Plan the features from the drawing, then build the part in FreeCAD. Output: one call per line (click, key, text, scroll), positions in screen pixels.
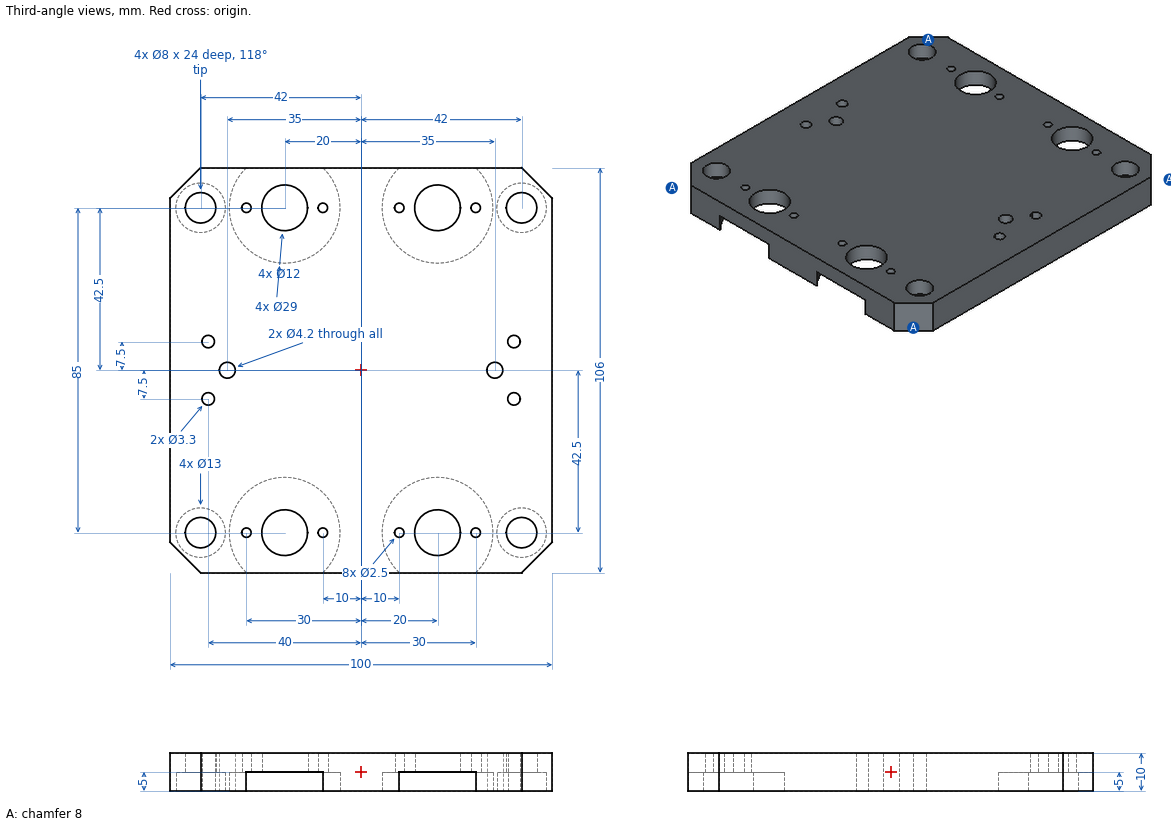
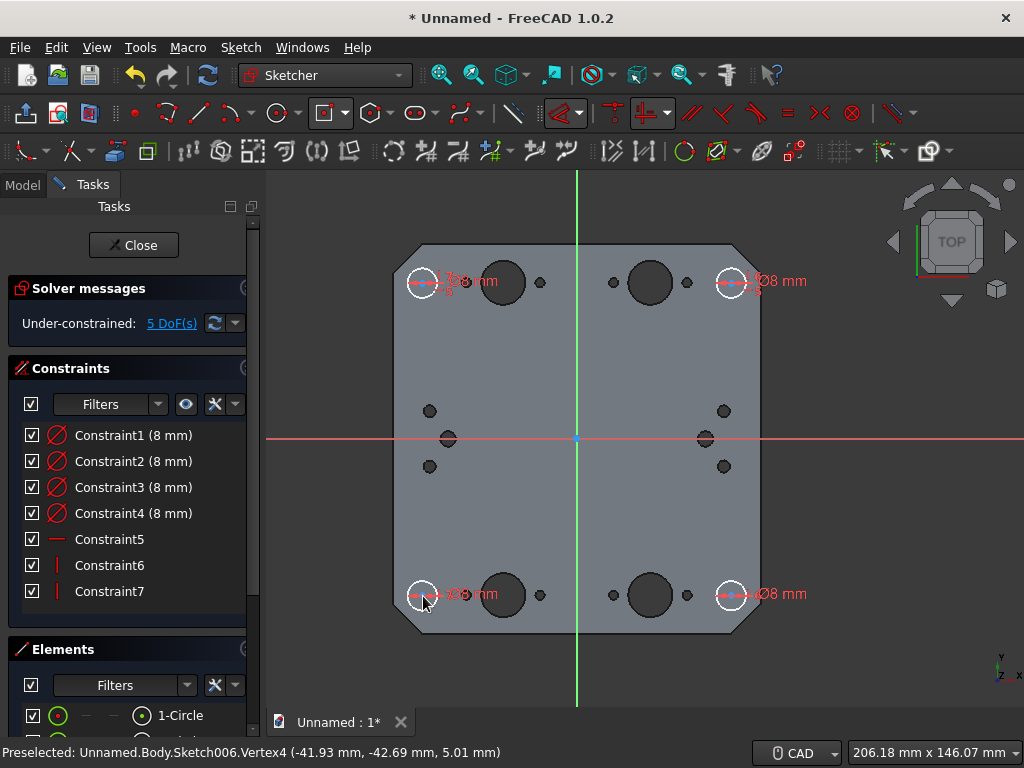
click(731, 596)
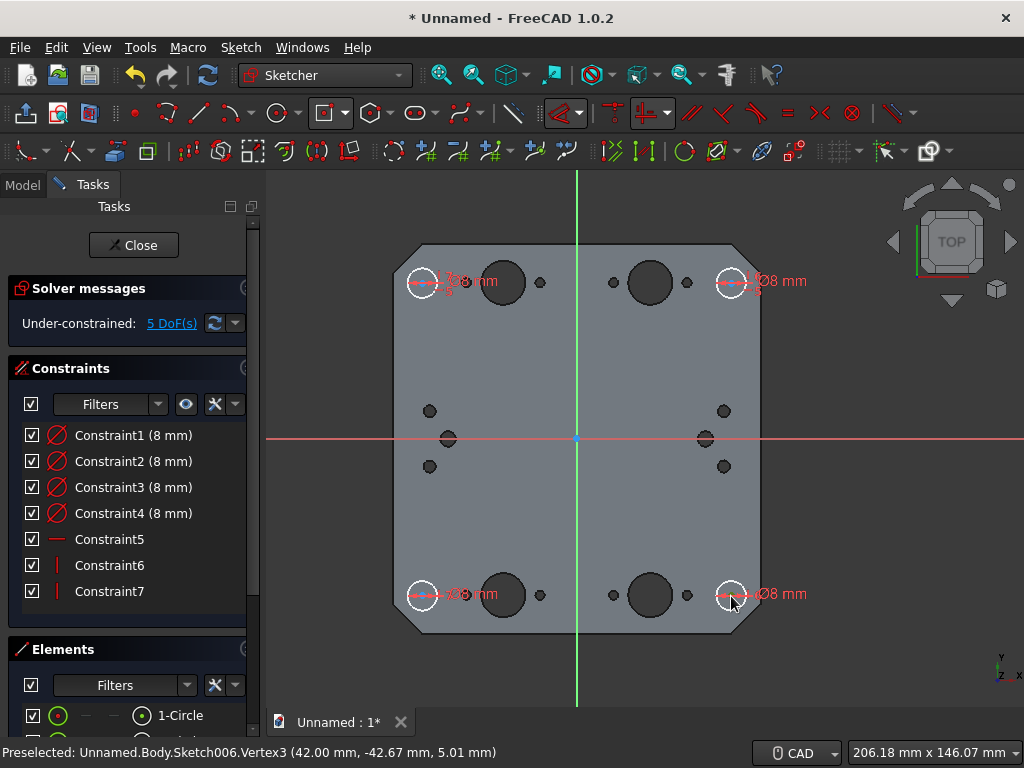
click(422, 596)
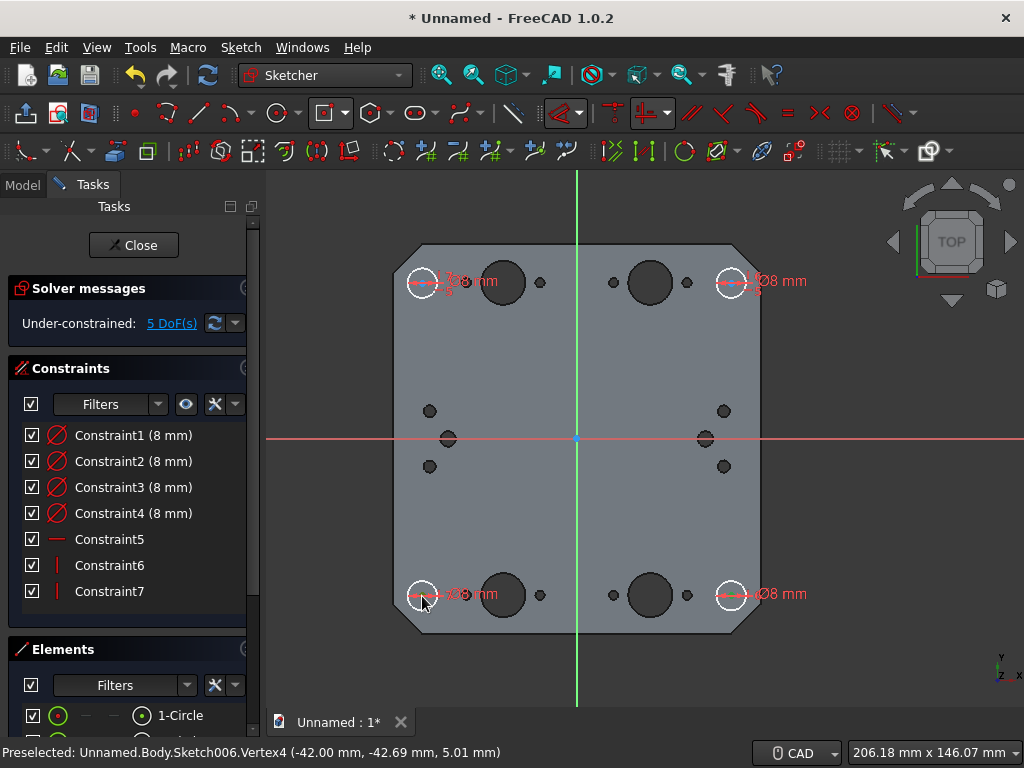
key(h)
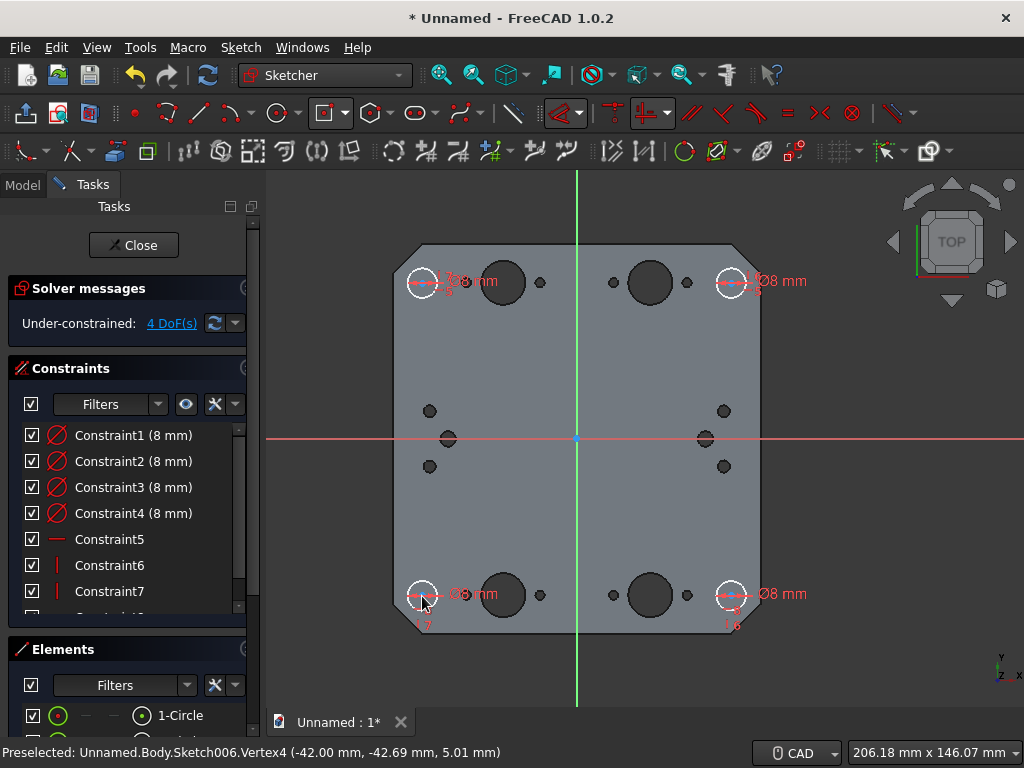
click(422, 283)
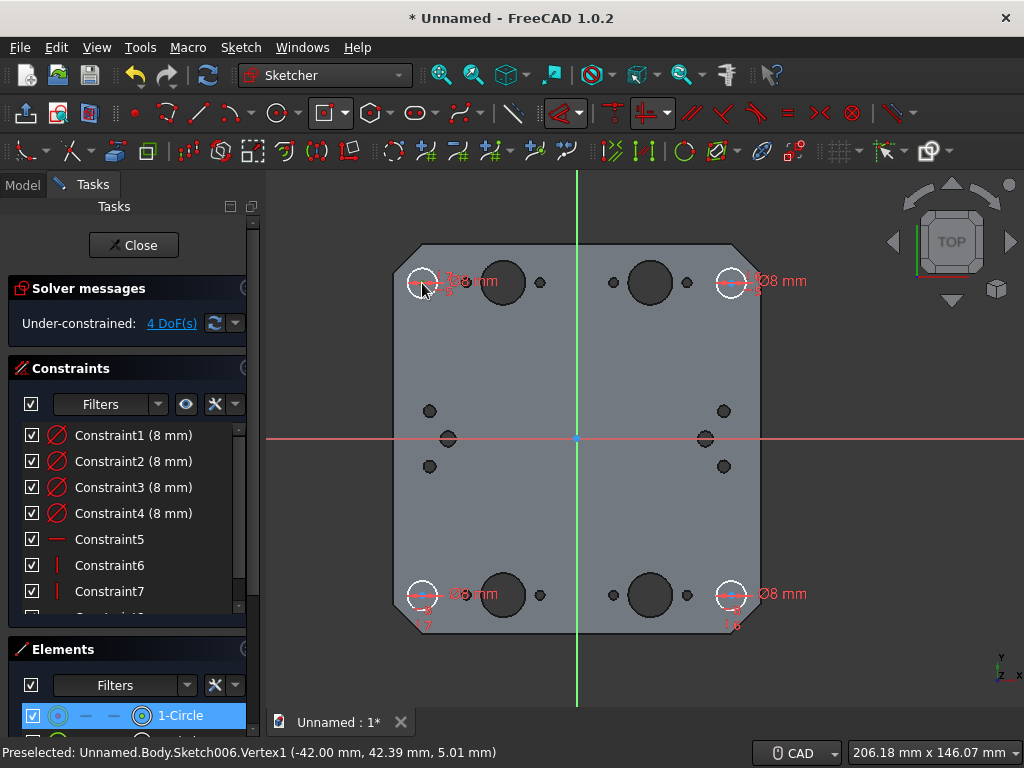
click(582, 114)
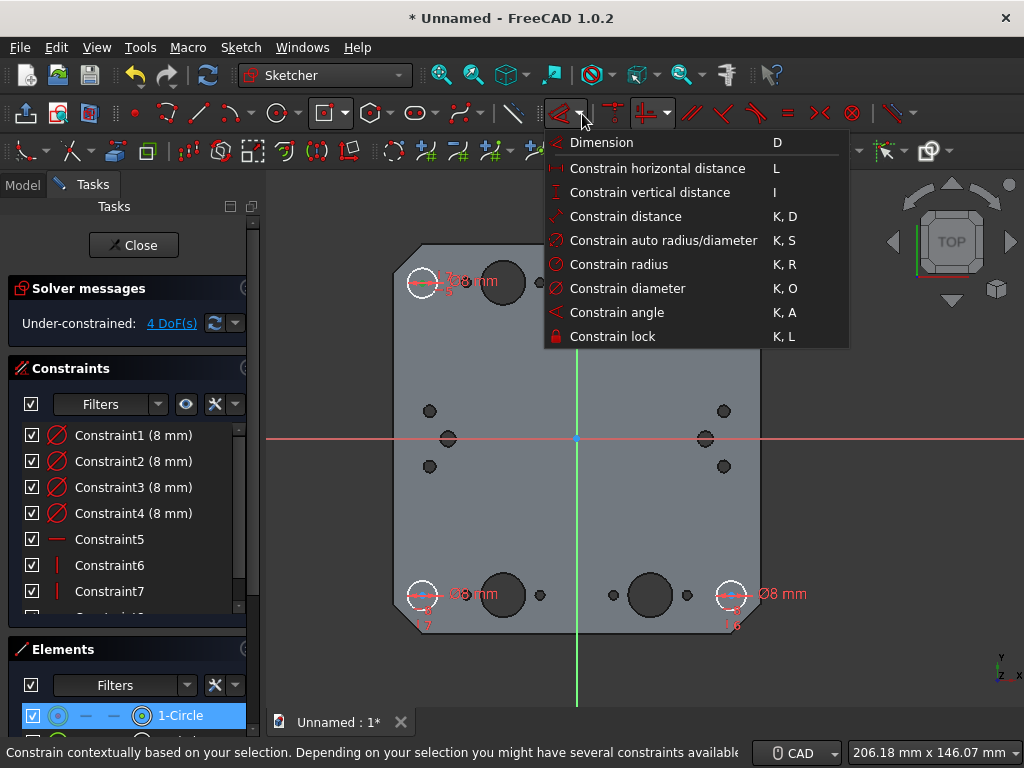
click(697, 168)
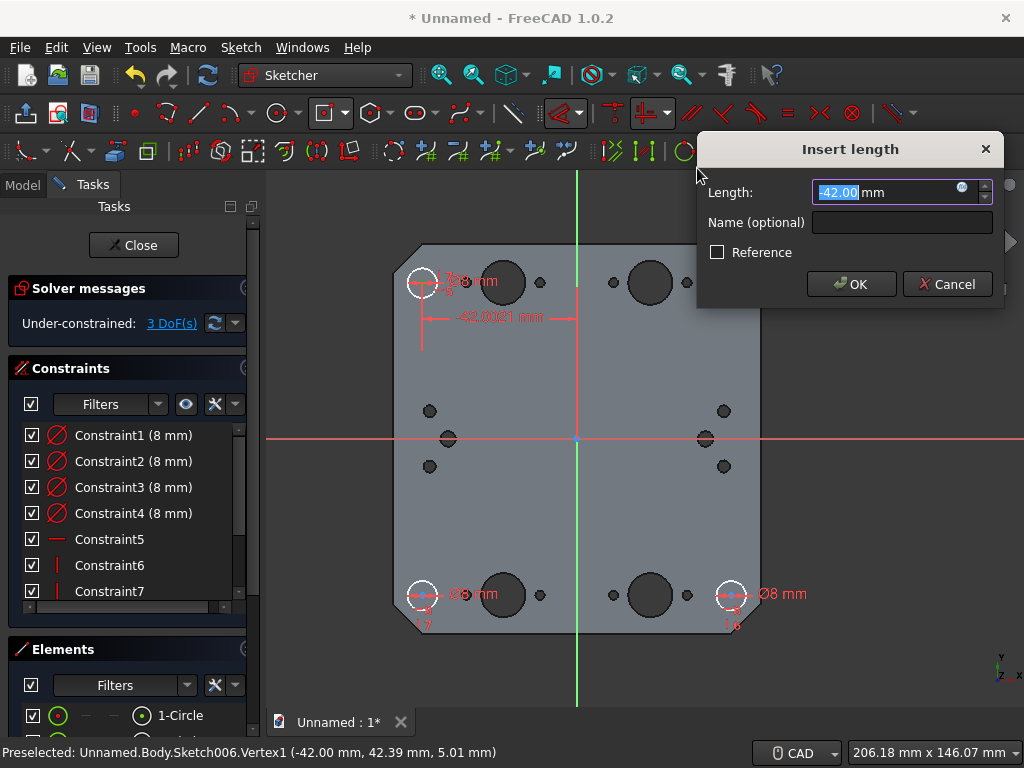
text(-42)
key(Return)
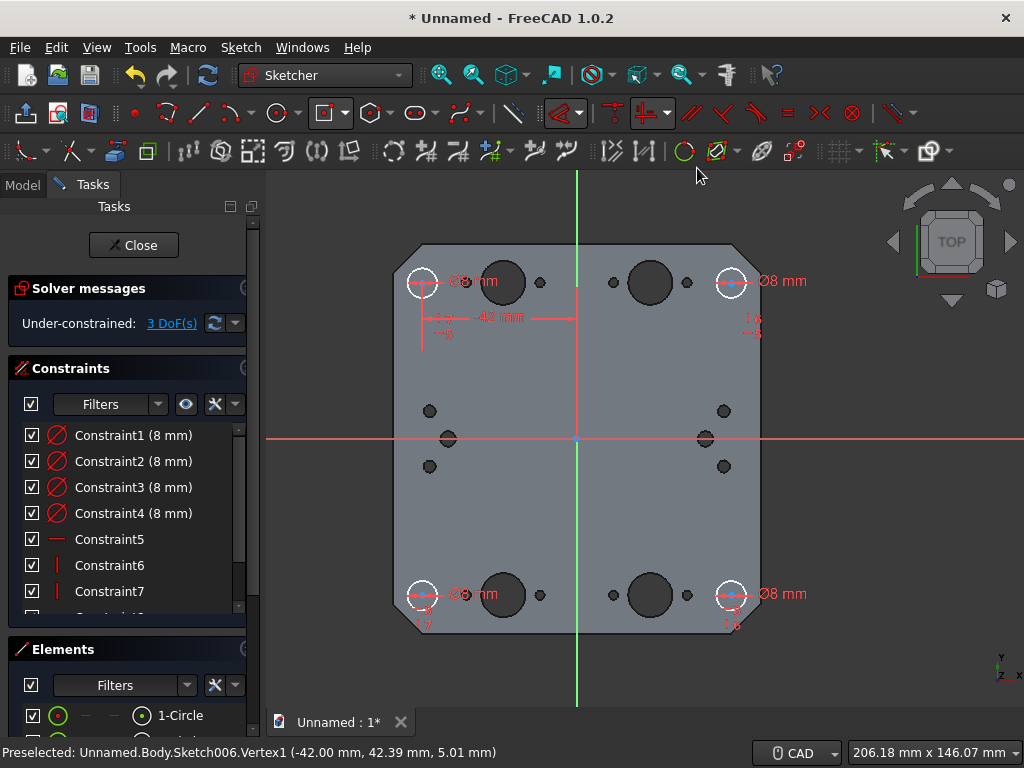
click(731, 283)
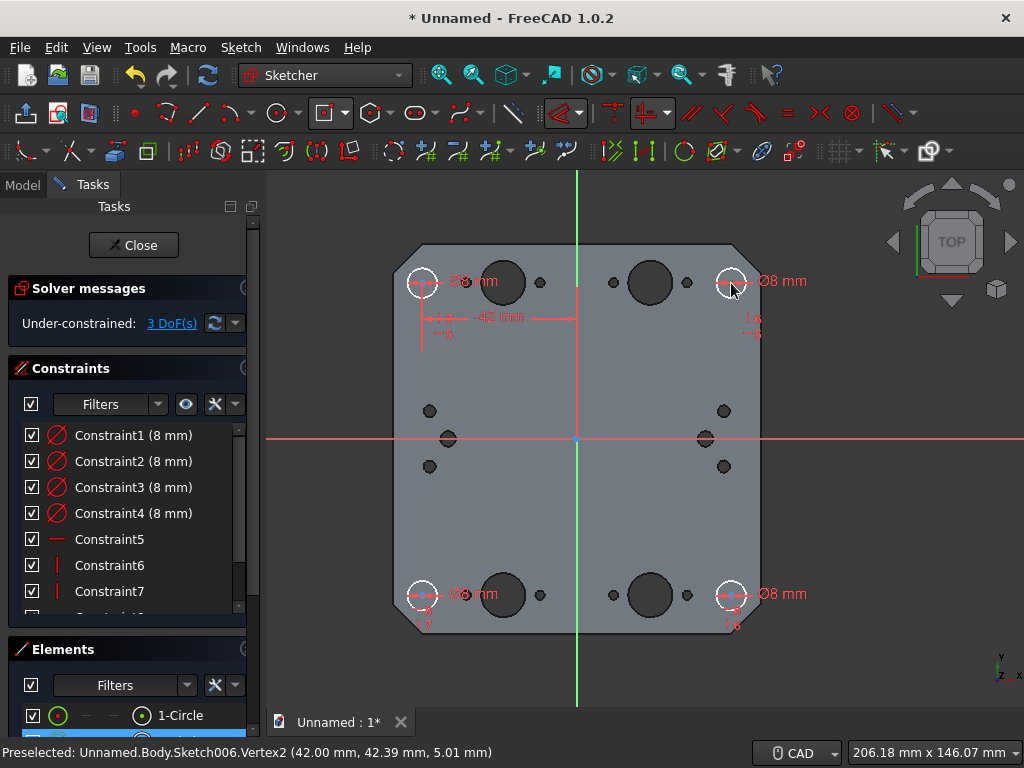
click(582, 114)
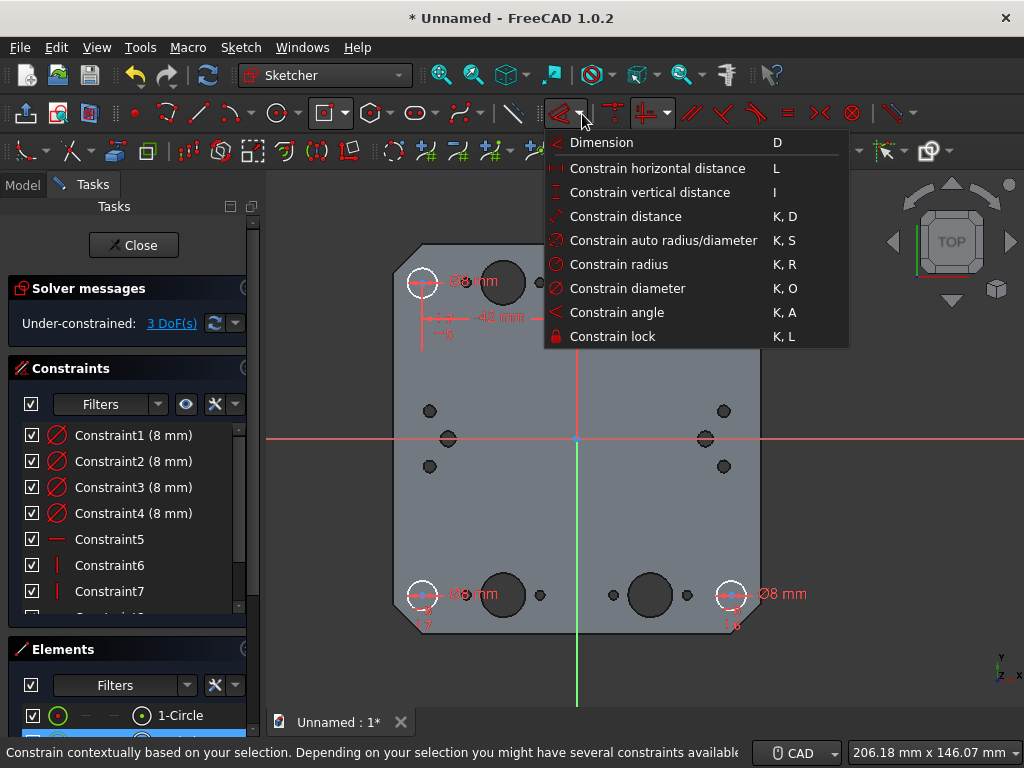
click(697, 168)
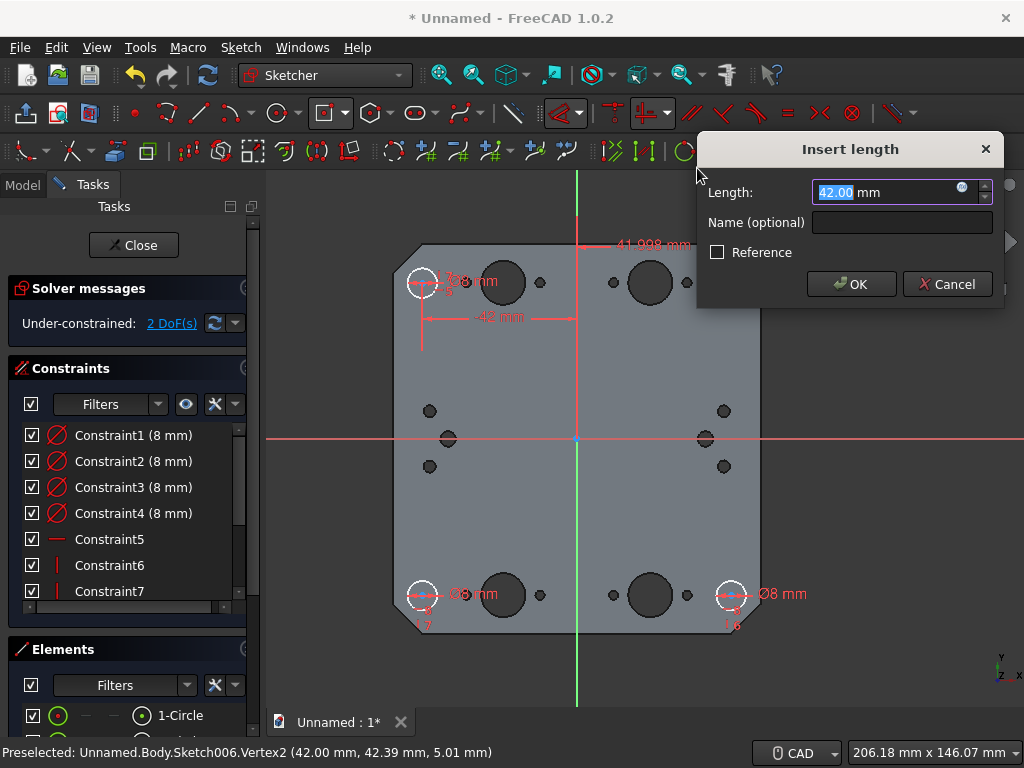
text(42)
key(Return)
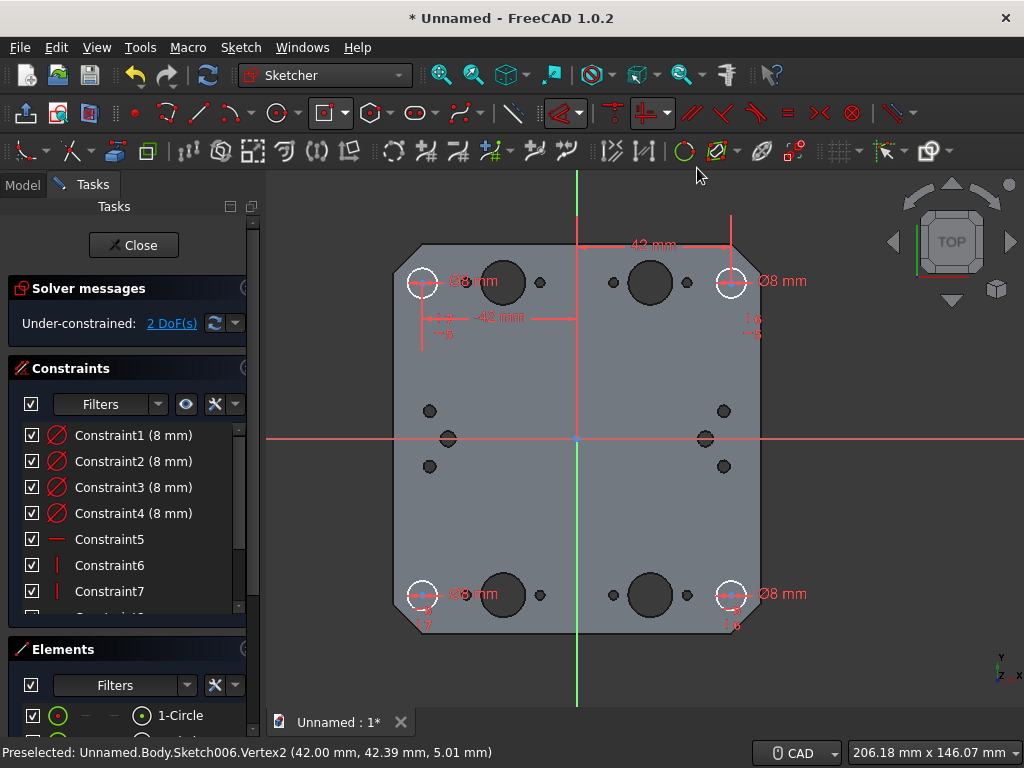
click(731, 283)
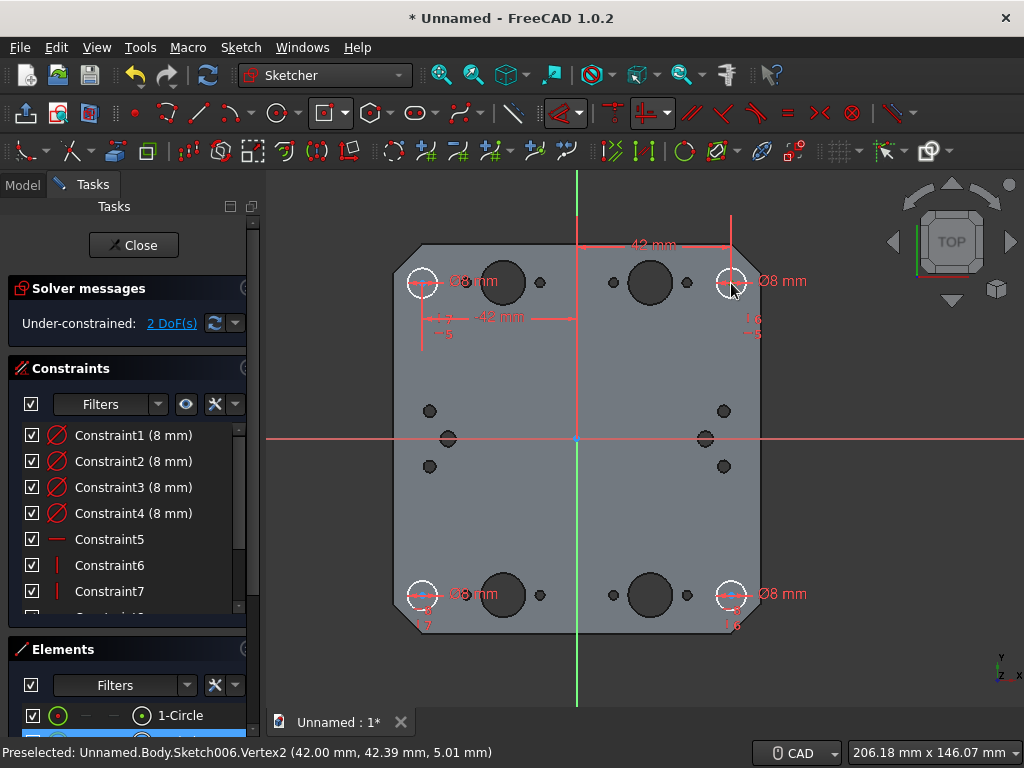
click(731, 596)